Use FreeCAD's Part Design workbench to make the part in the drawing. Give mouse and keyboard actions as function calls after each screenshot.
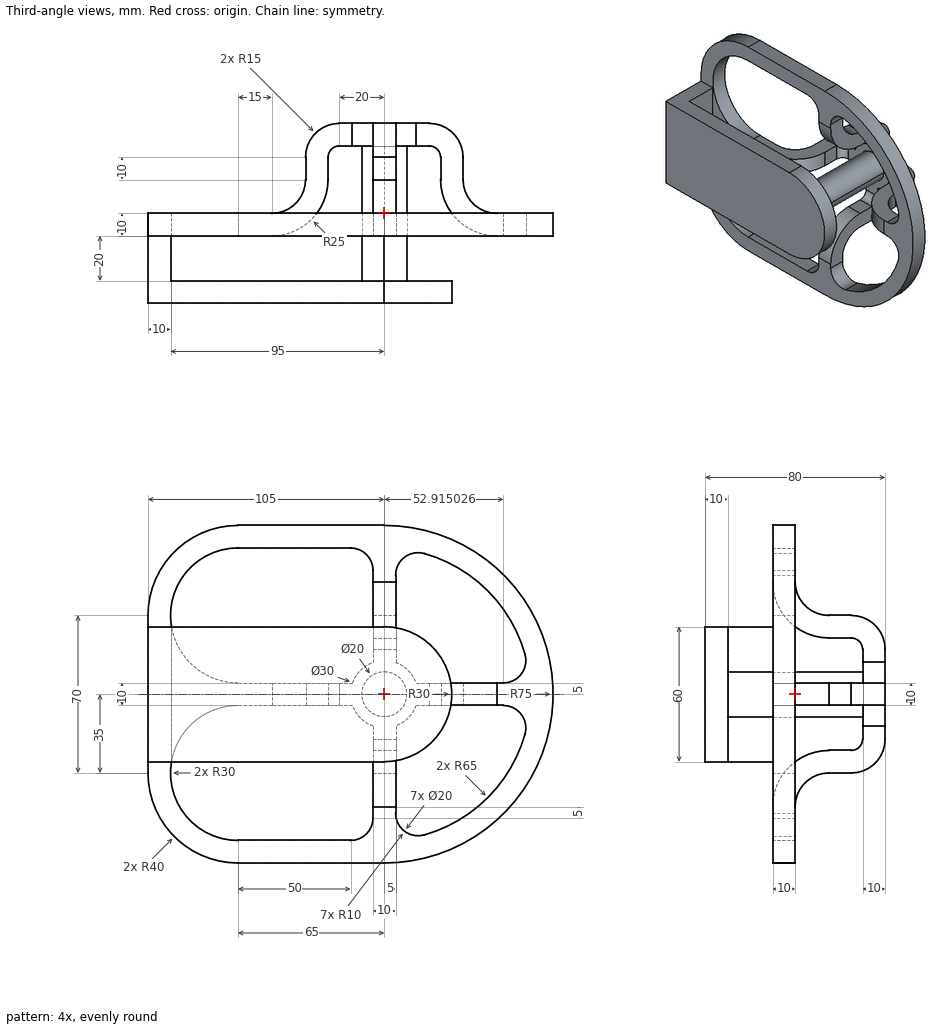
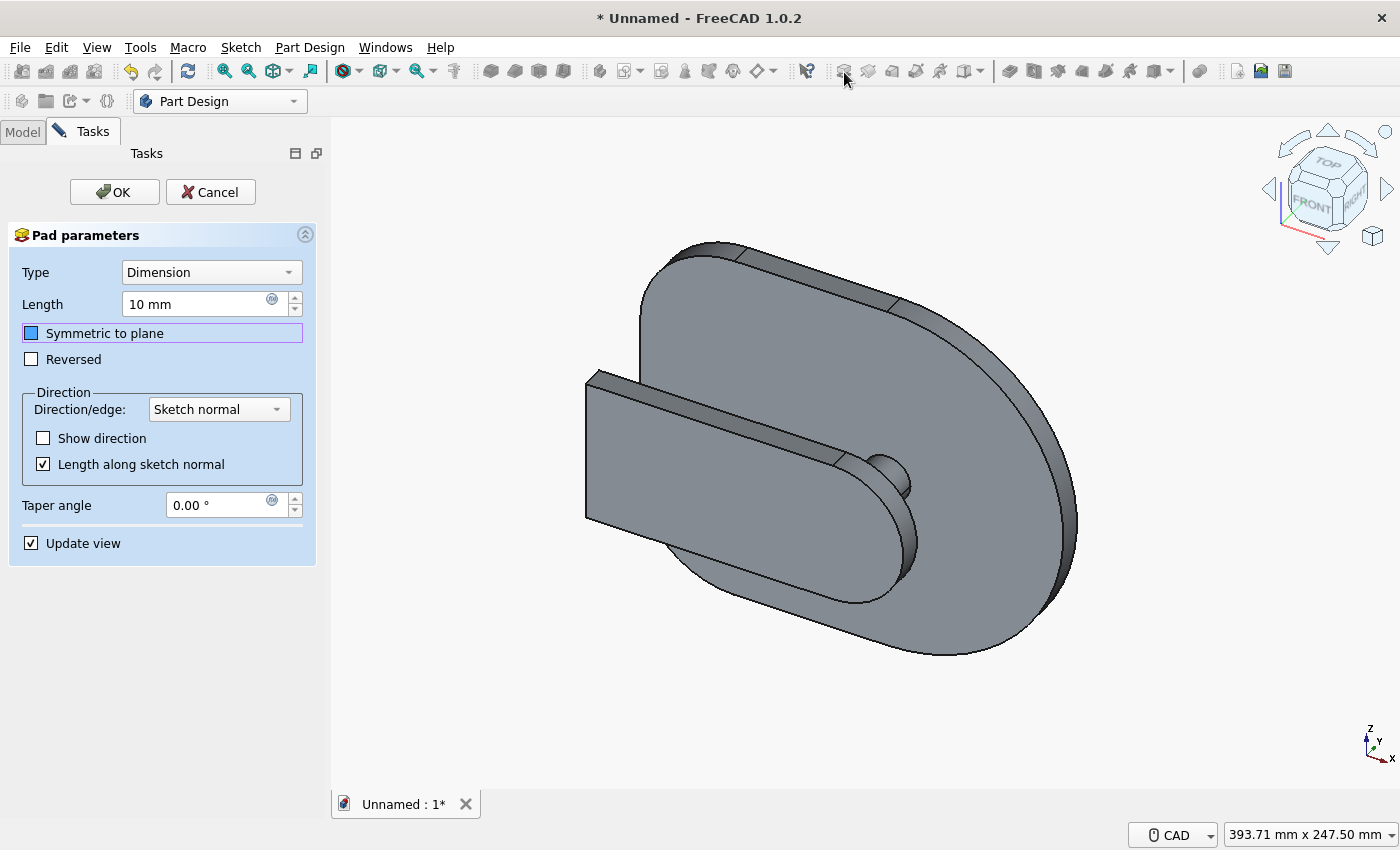
click(30, 359)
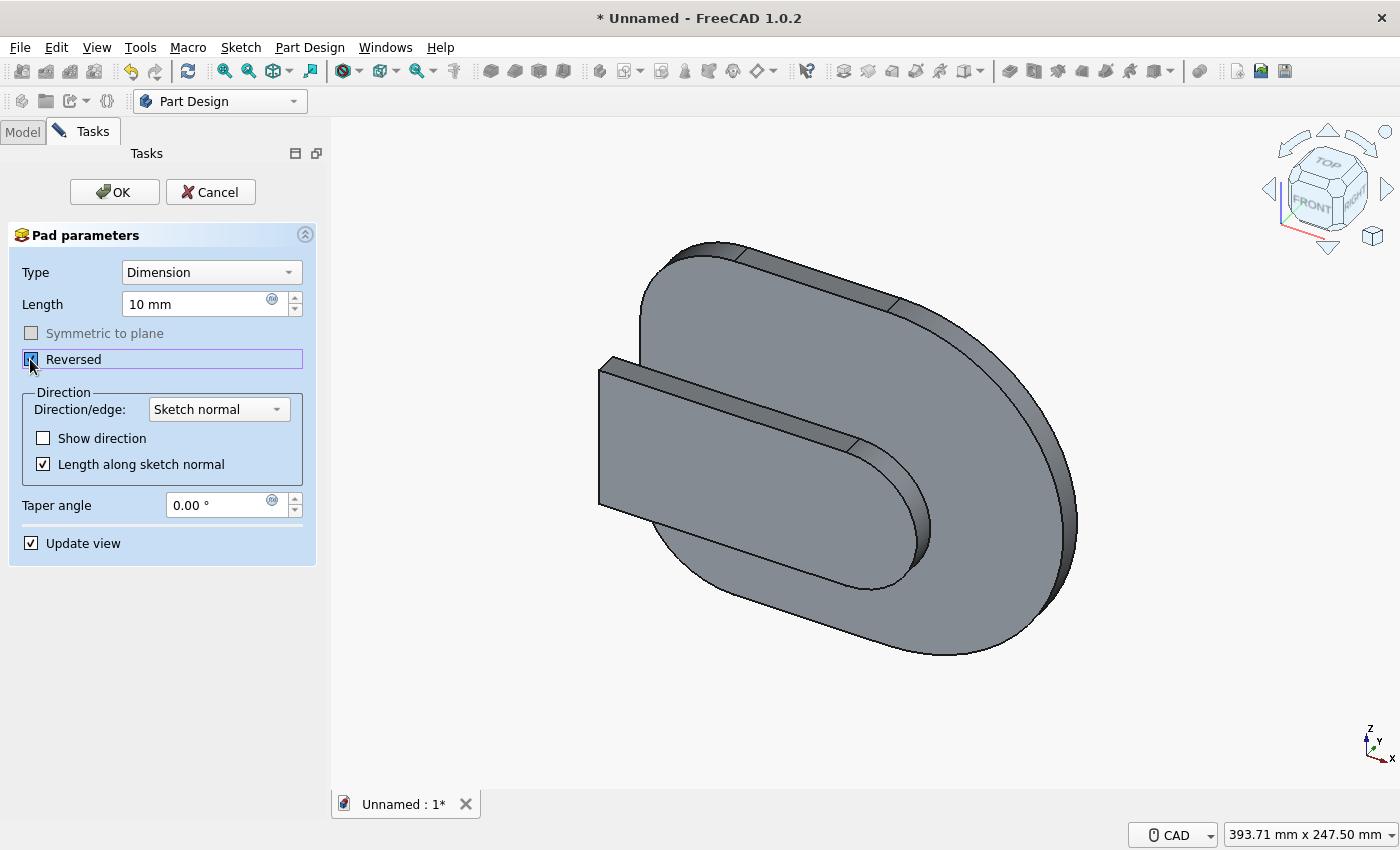
click(115, 192)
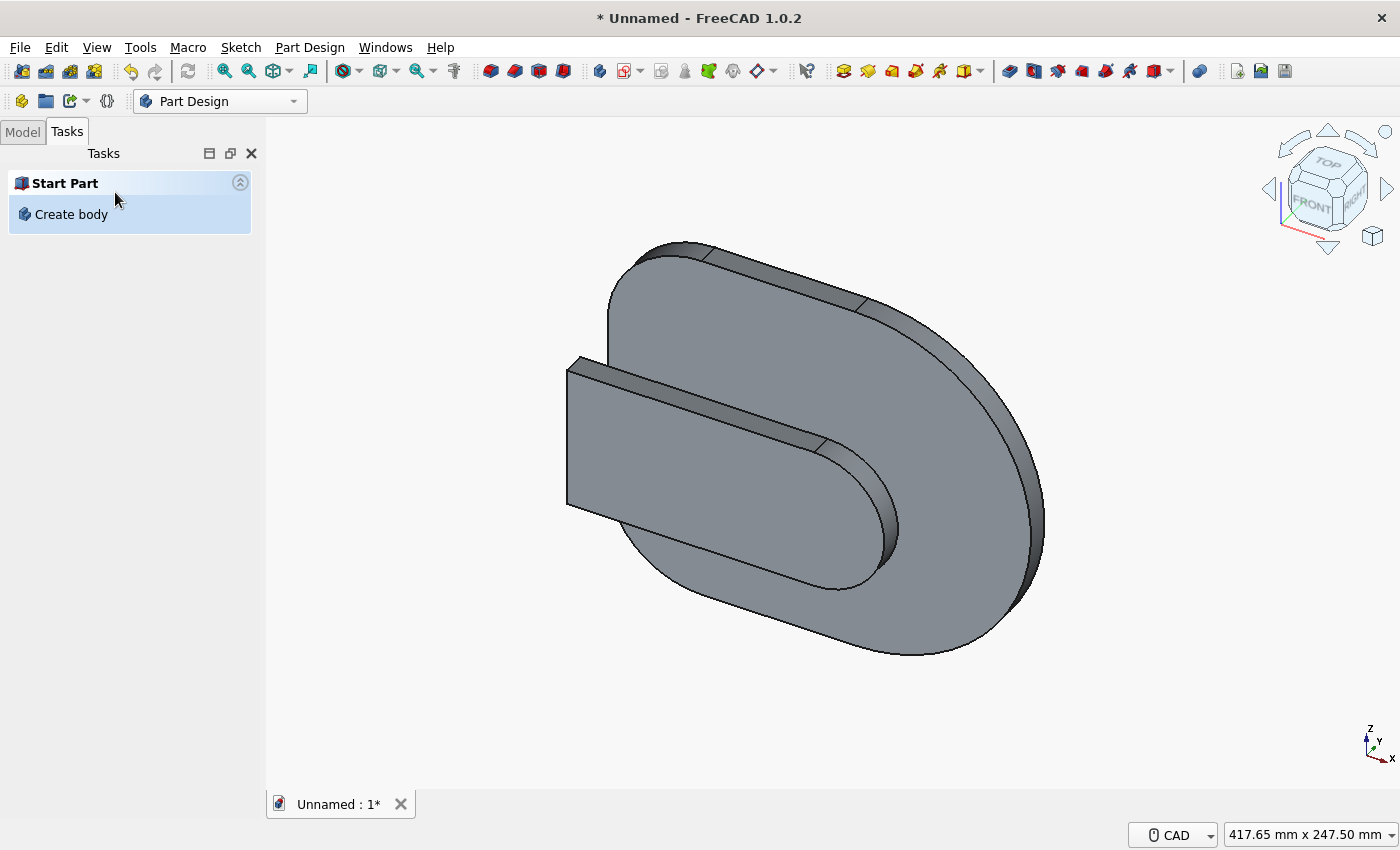
click(624, 72)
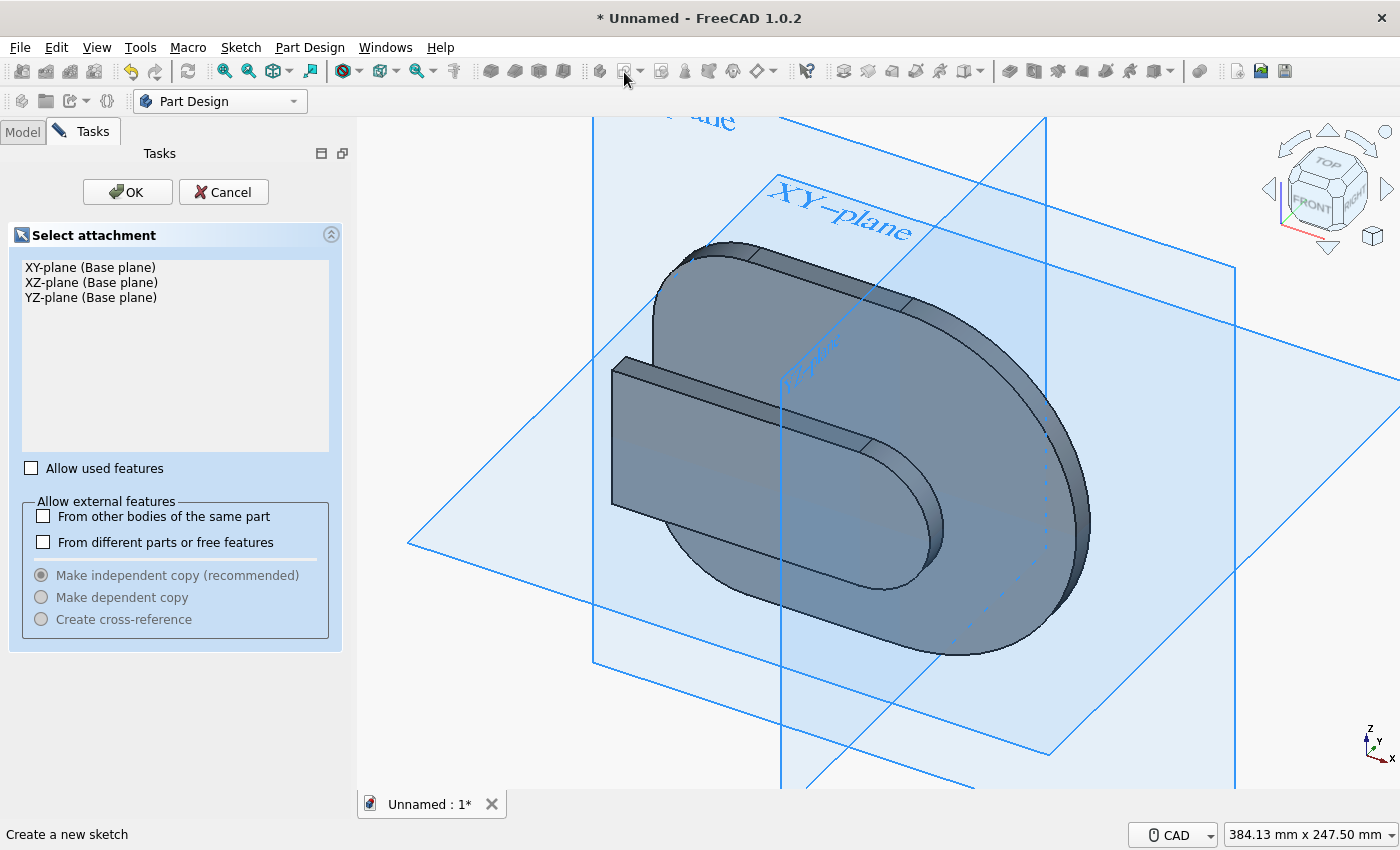
click(82, 268)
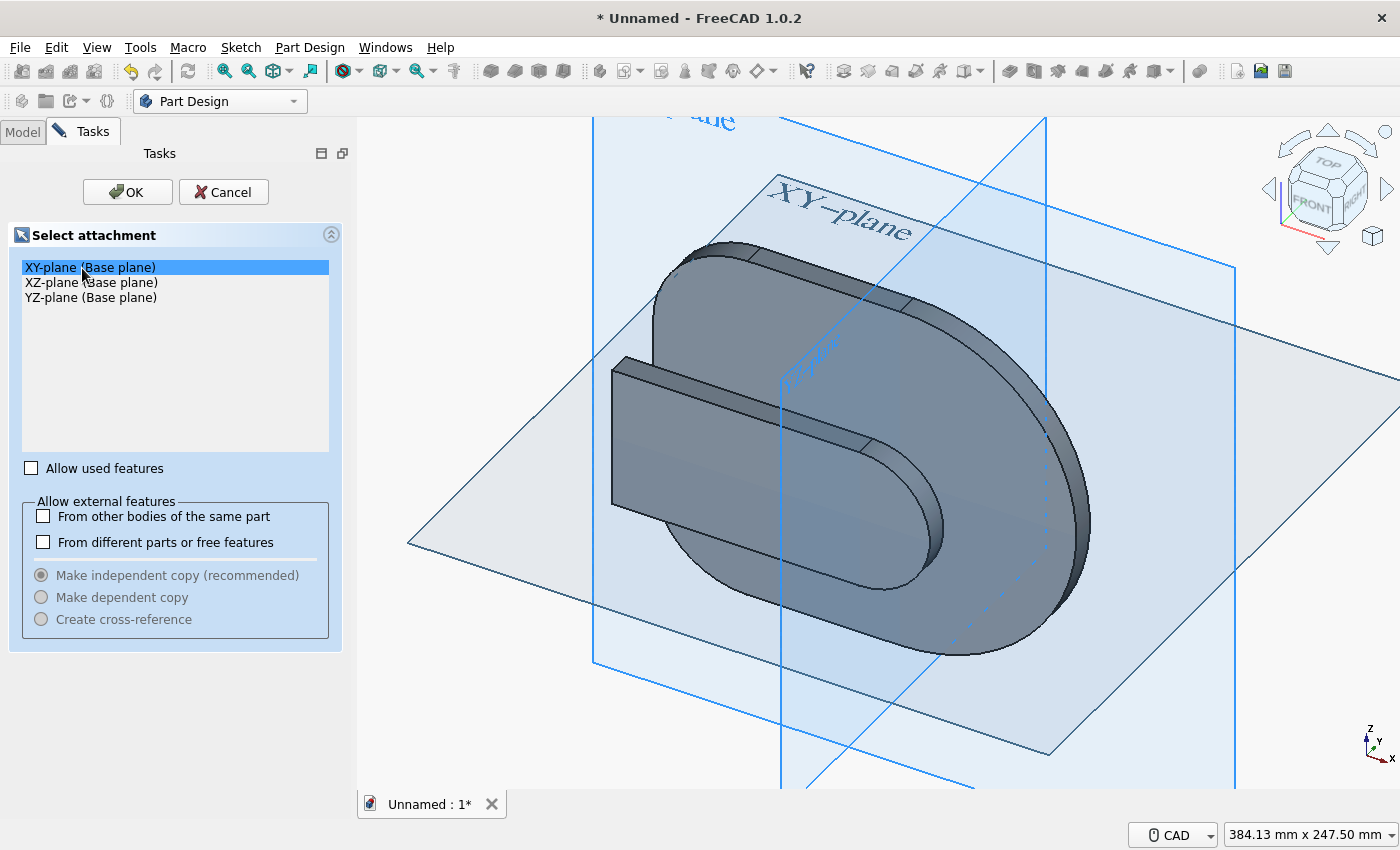
click(128, 192)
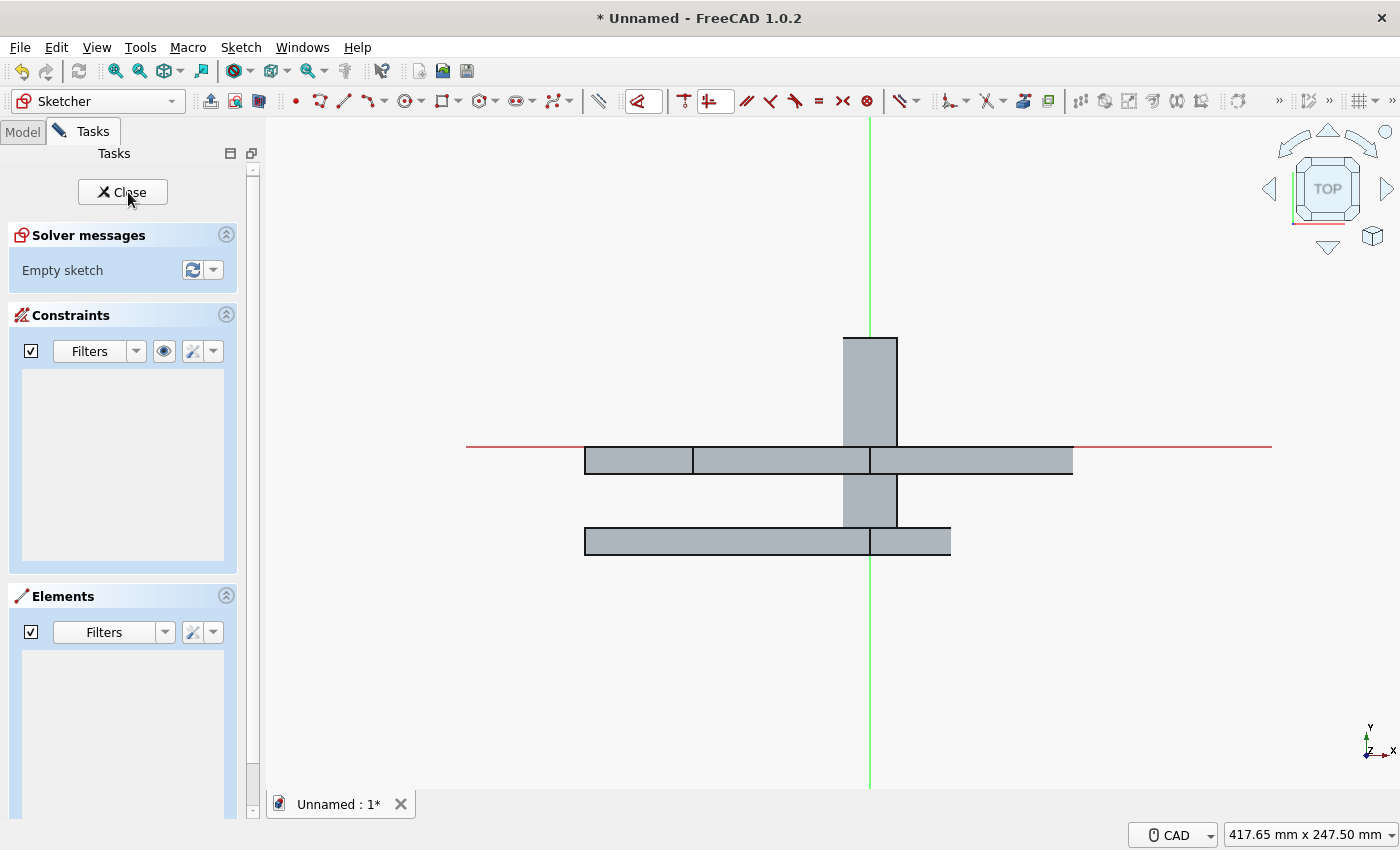
click(260, 102)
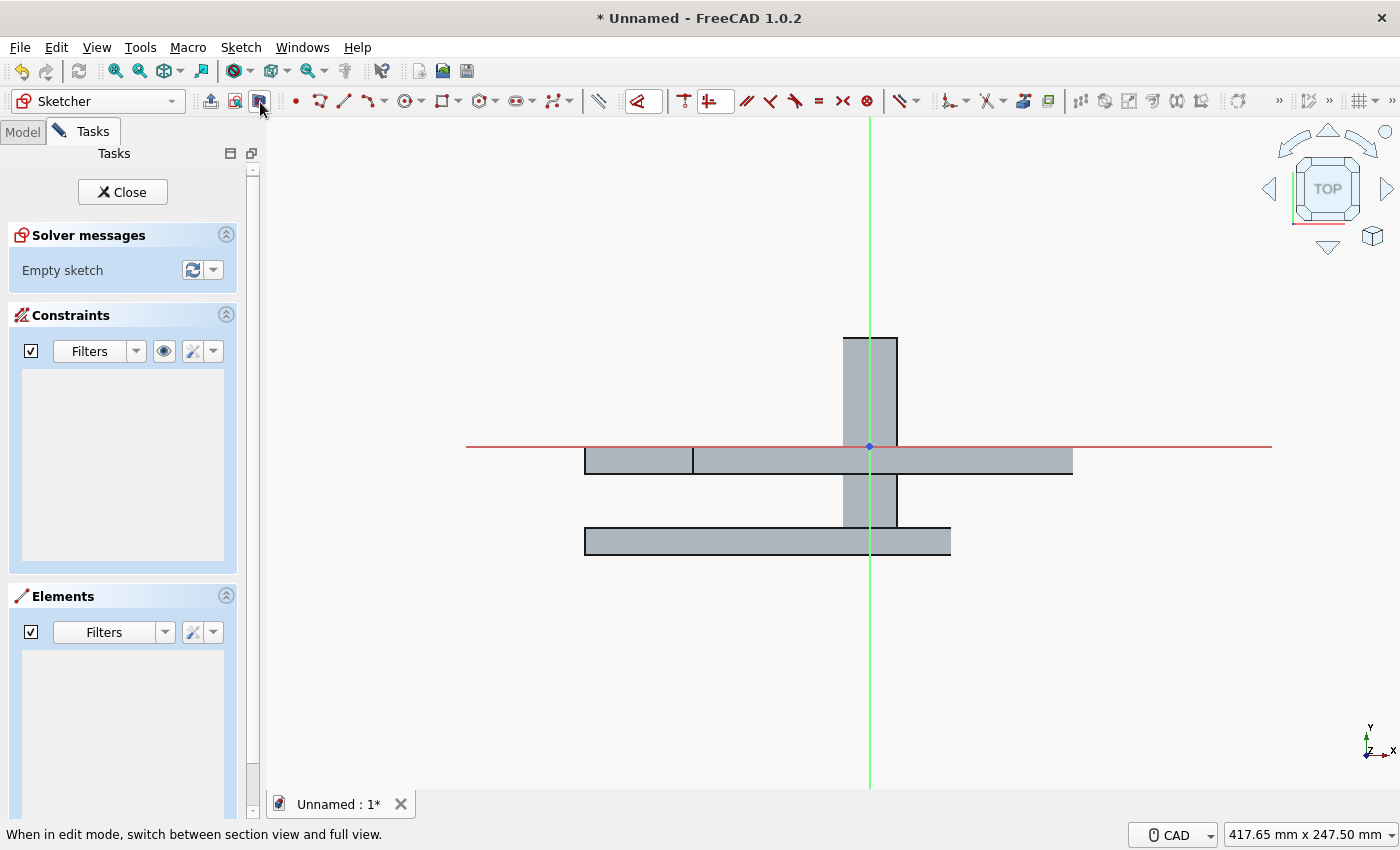
scroll(572, 508, up, 10)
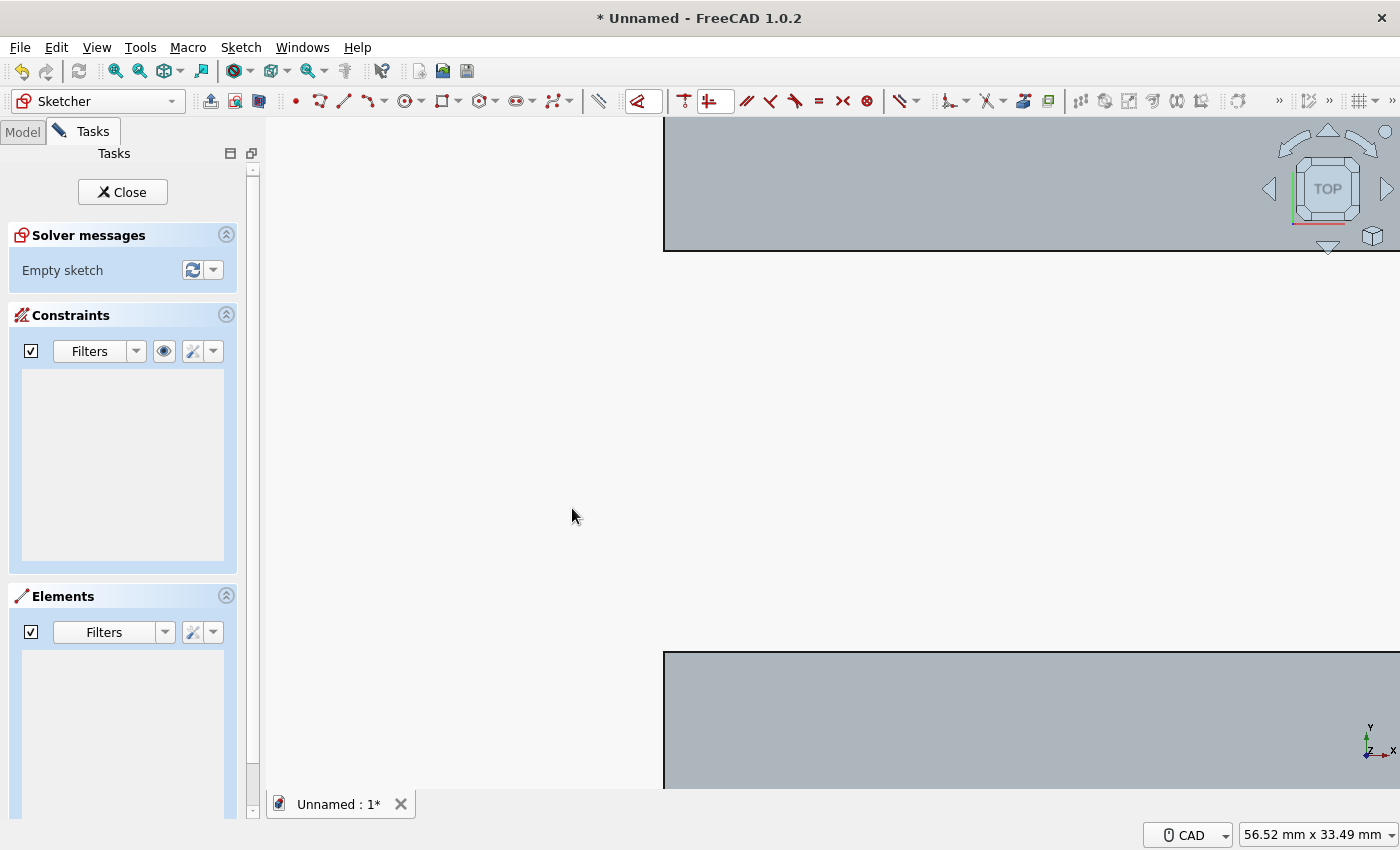
click(442, 102)